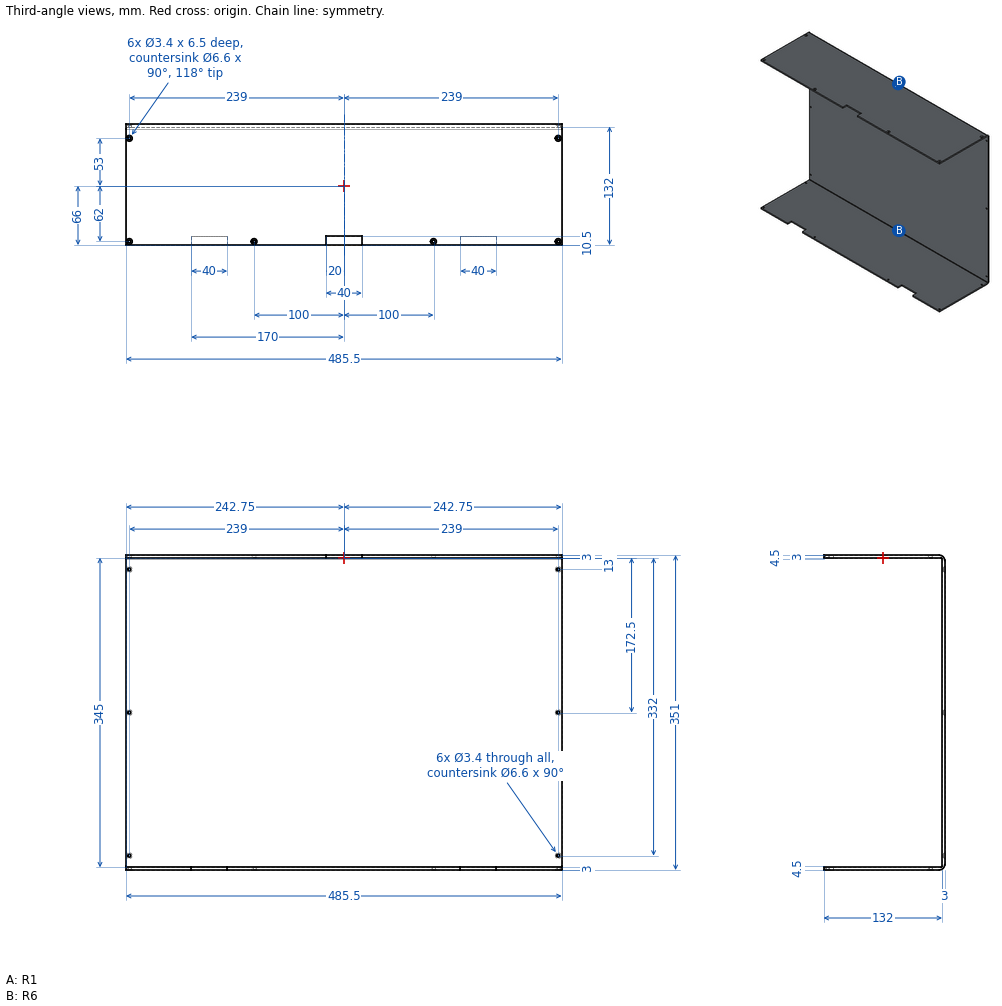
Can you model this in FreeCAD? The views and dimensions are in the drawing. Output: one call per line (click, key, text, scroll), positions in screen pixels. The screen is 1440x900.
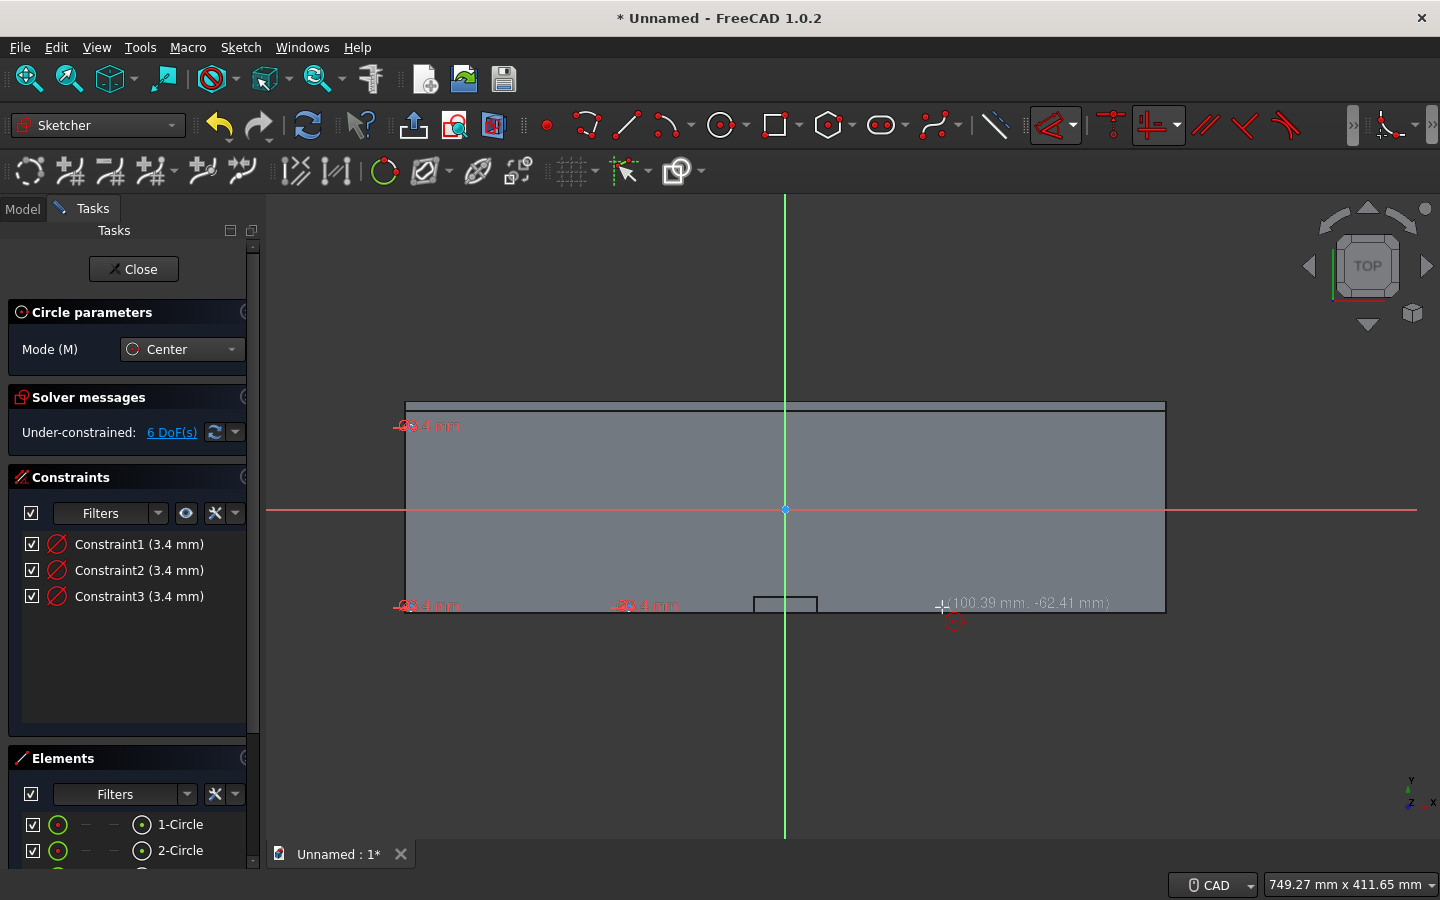
click(942, 607)
move(944, 605)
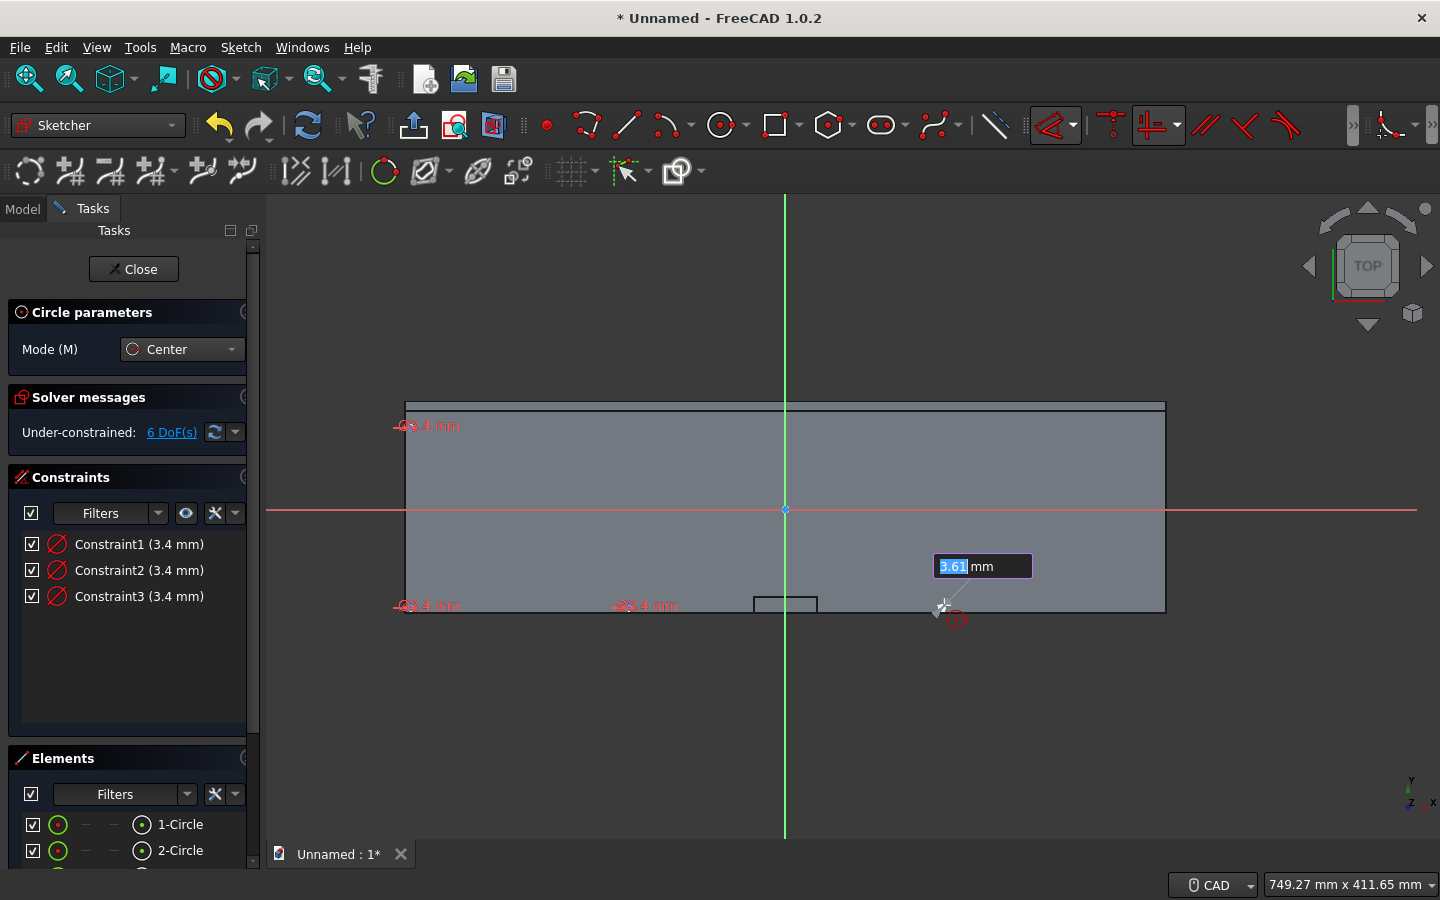
text(3.4)
key(Return)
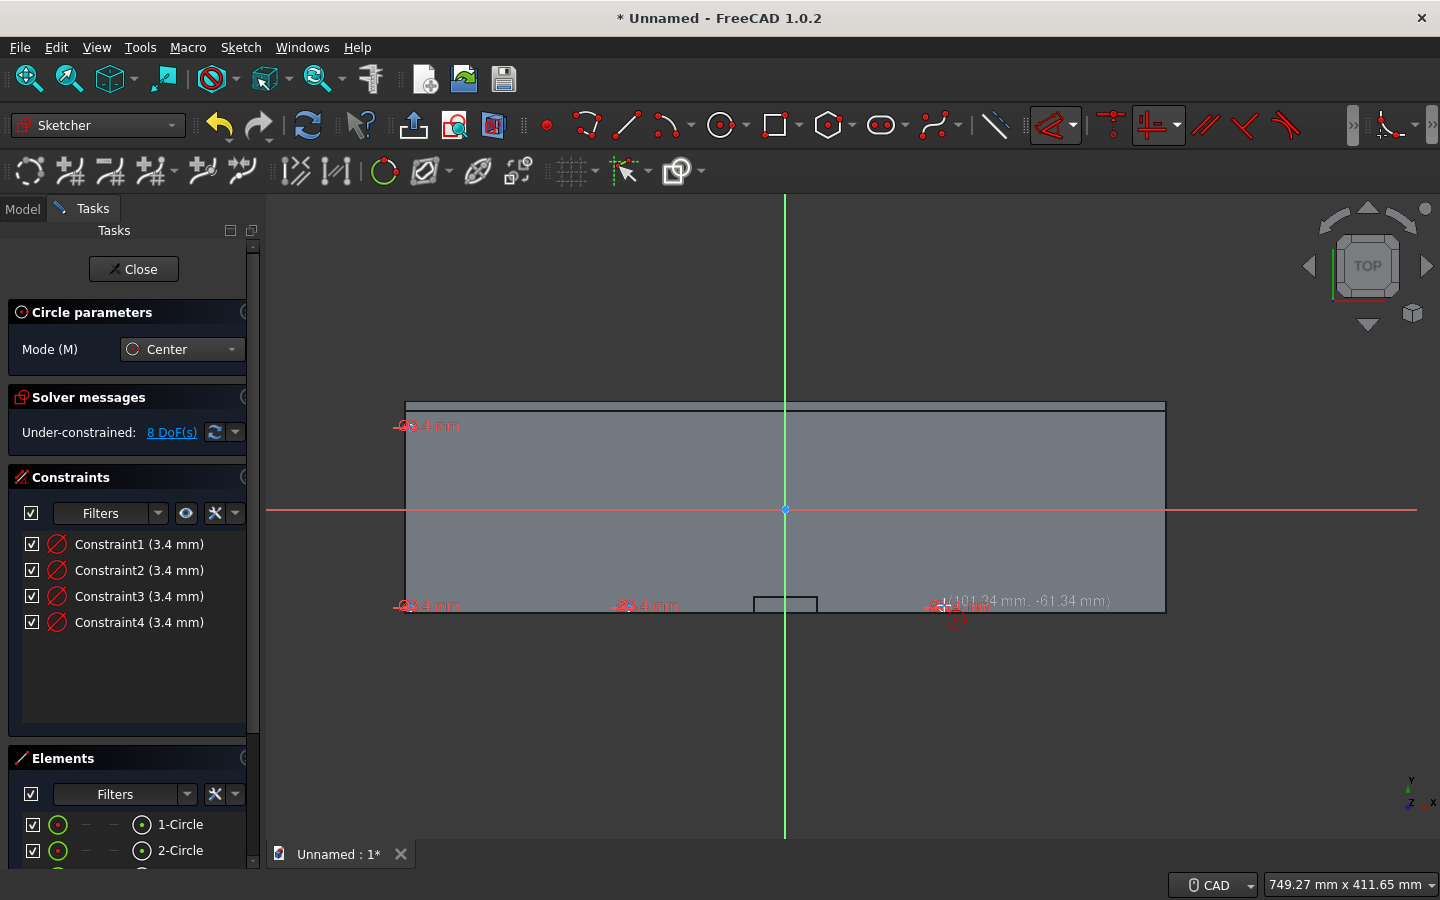
scroll(1160, 427, up, 11)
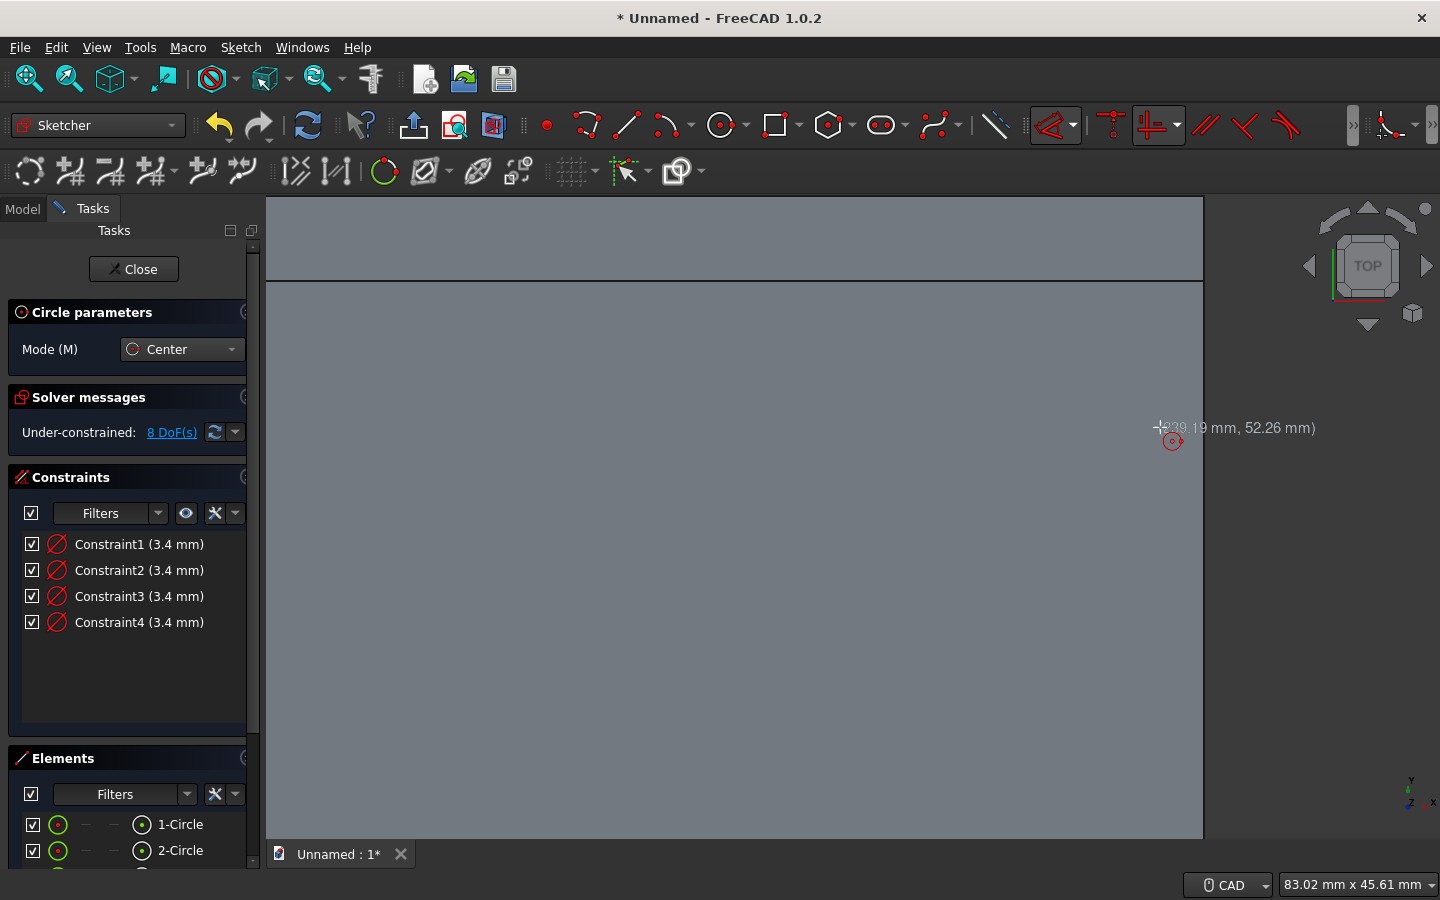
scroll(1160, 427, down, 11)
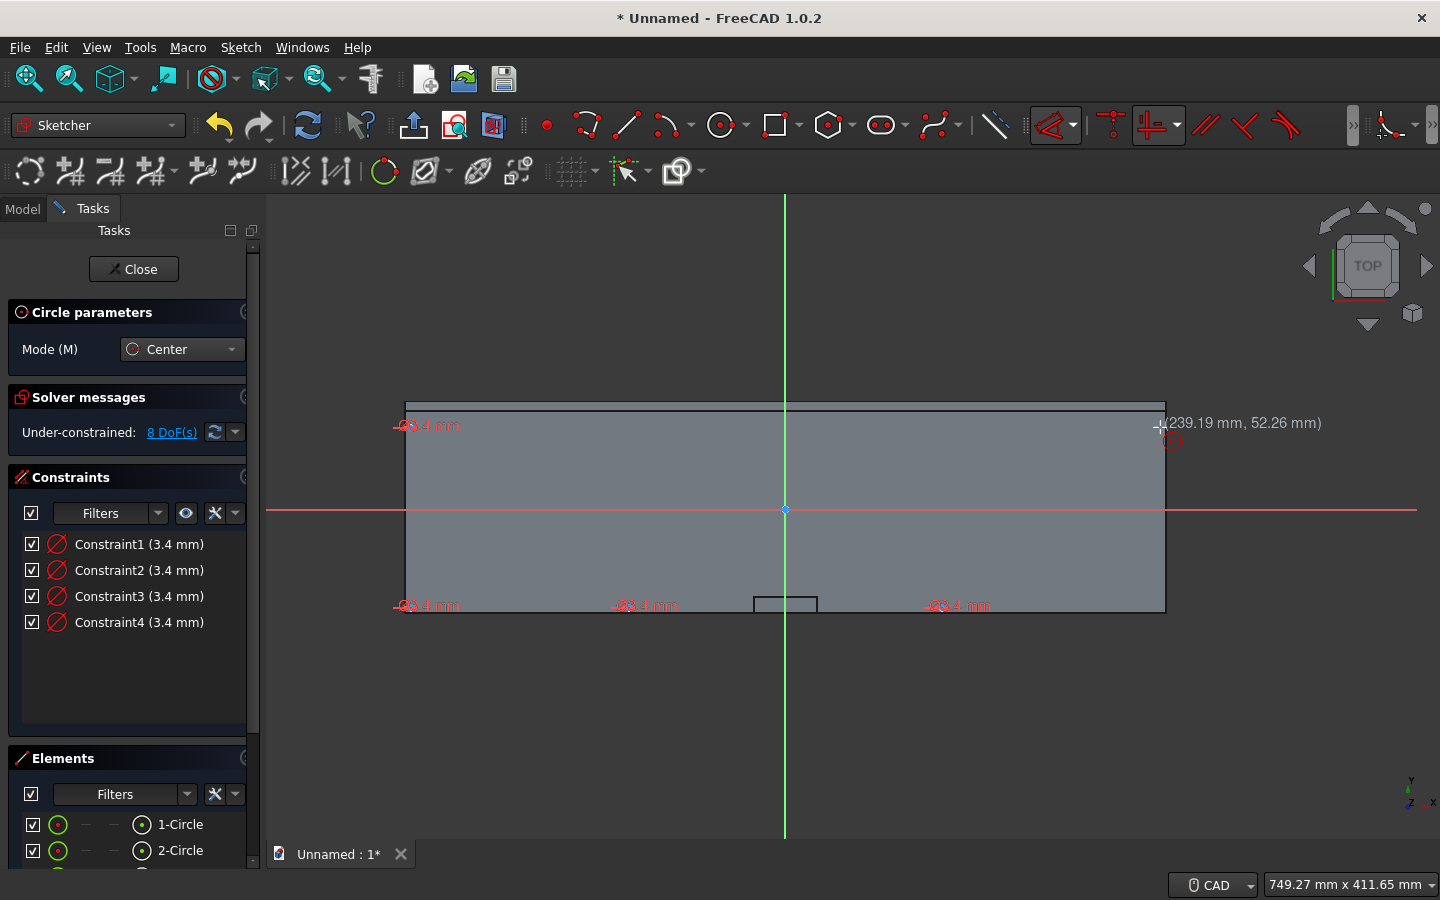
click(1160, 427)
move(1162, 425)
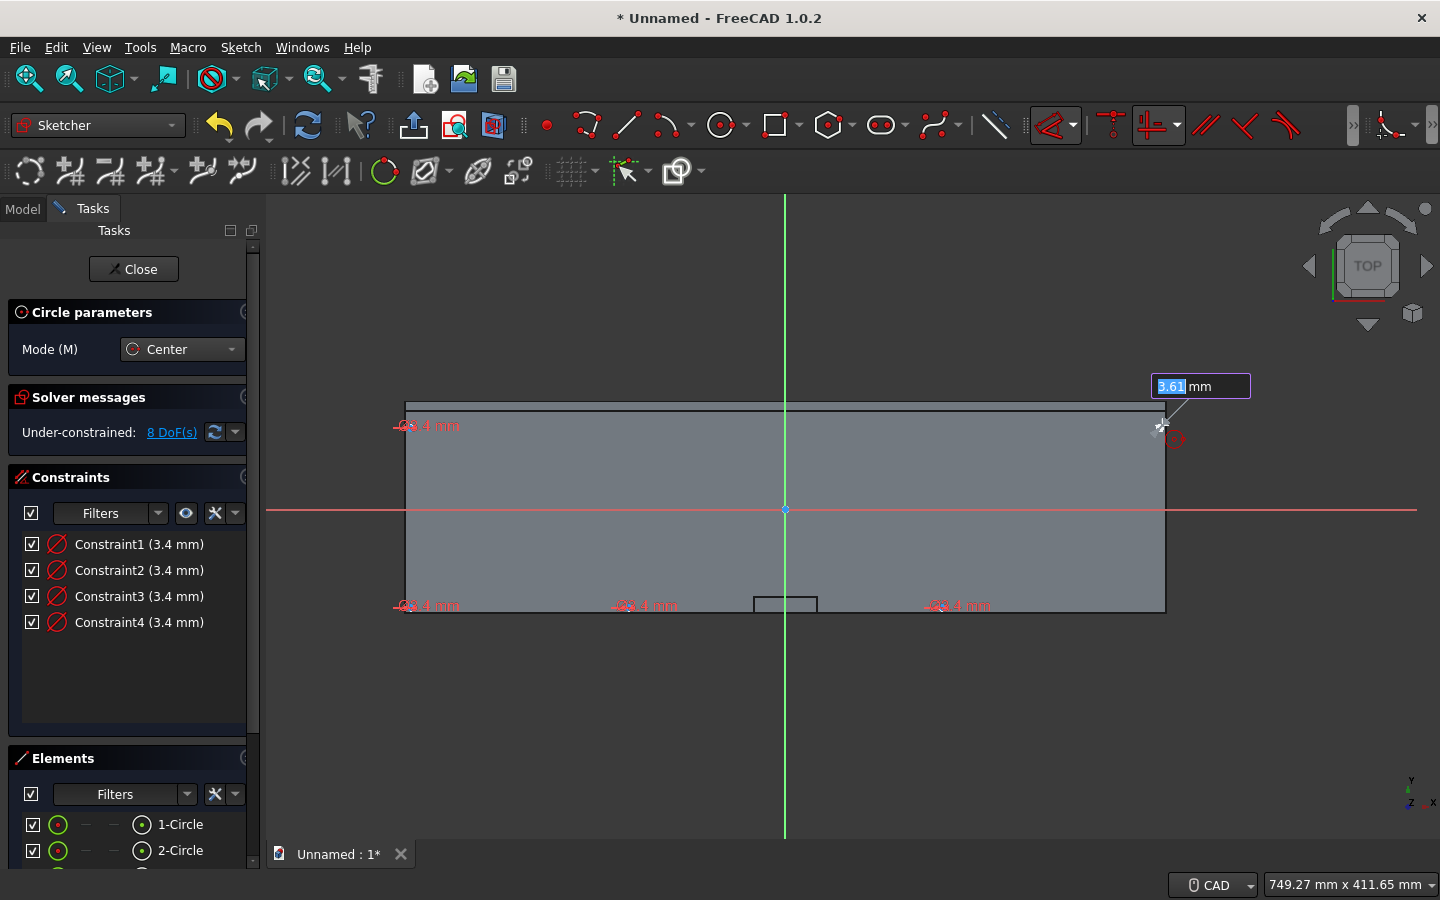
text(3.4)
key(Return)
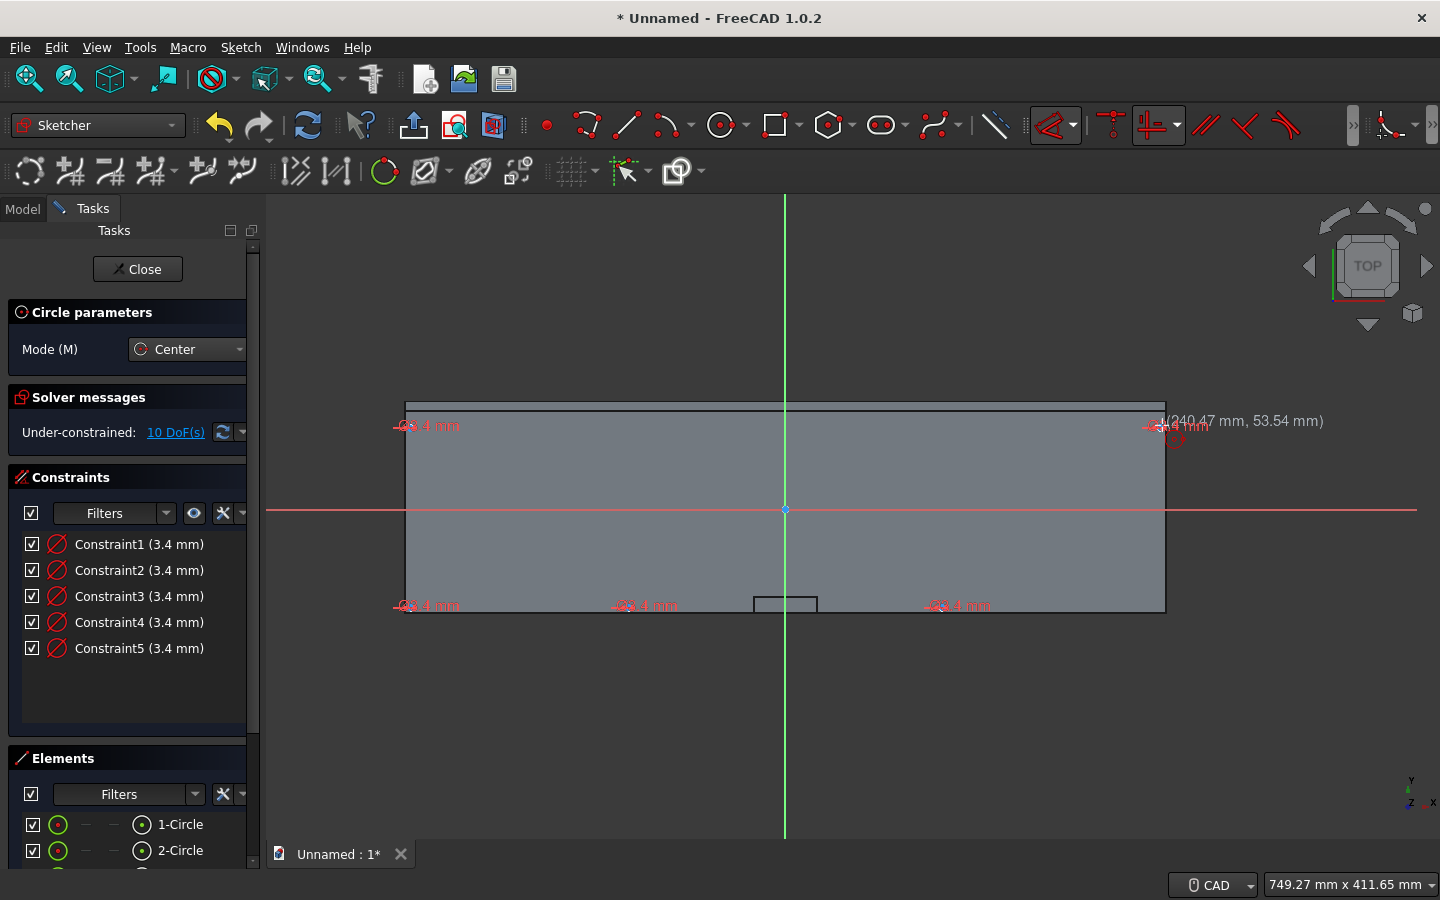
scroll(1160, 607, up, 11)